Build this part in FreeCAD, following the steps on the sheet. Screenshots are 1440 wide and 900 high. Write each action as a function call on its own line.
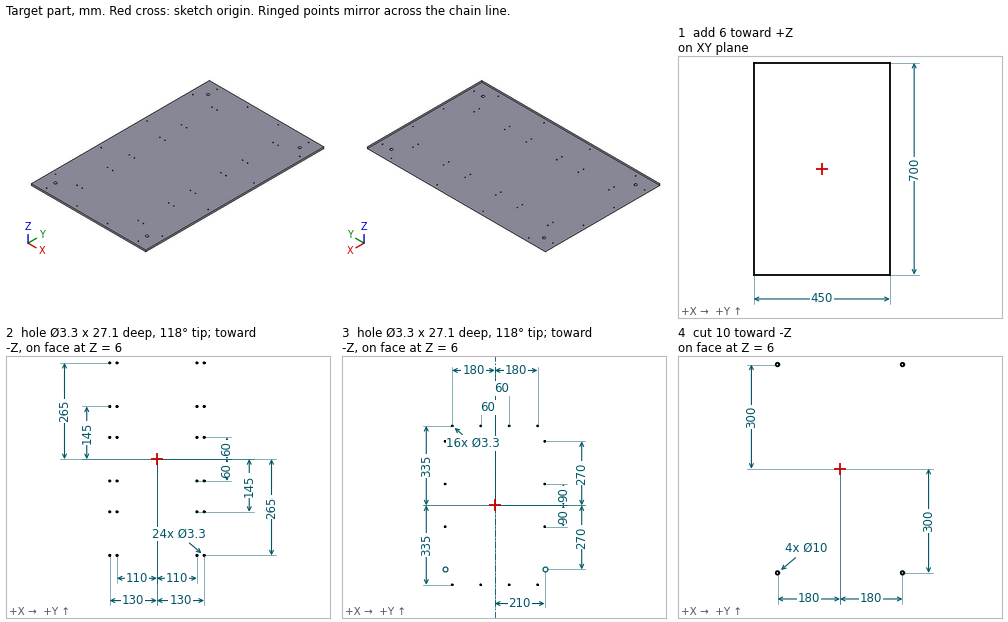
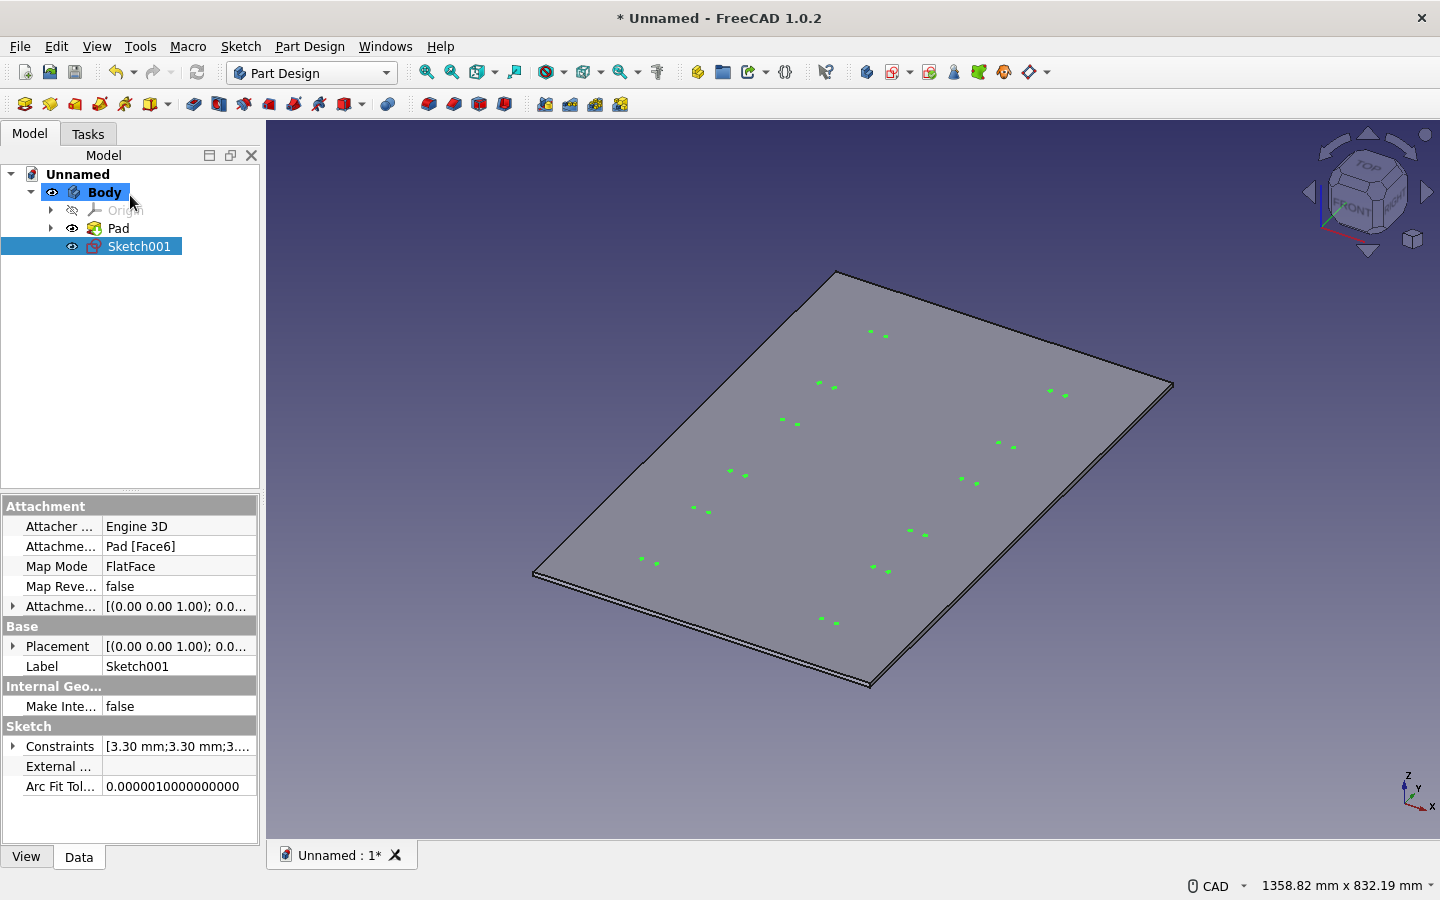
click(219, 104)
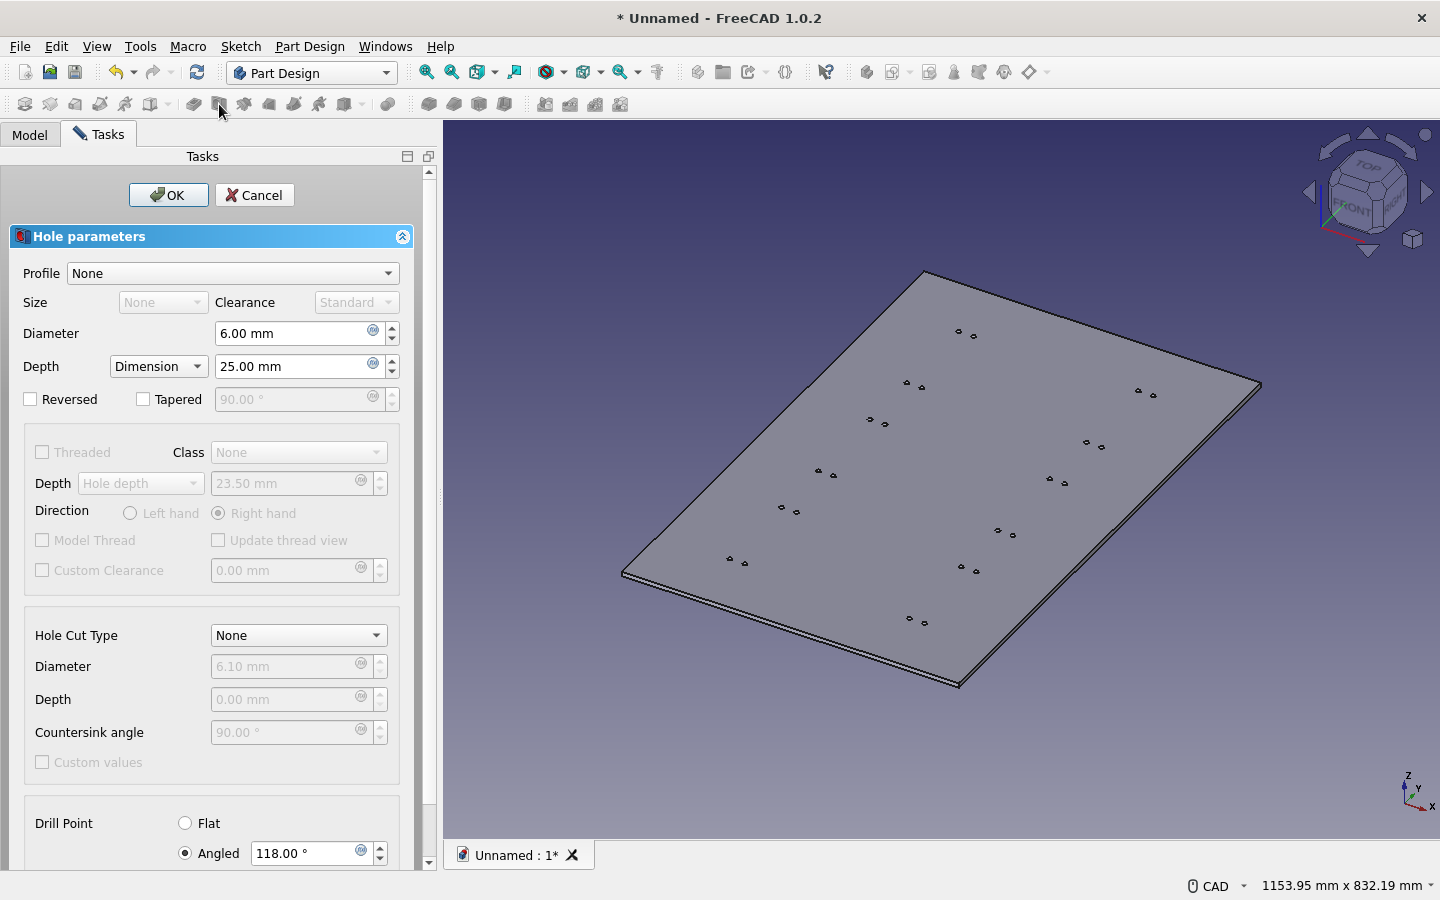
triple_click(300, 334)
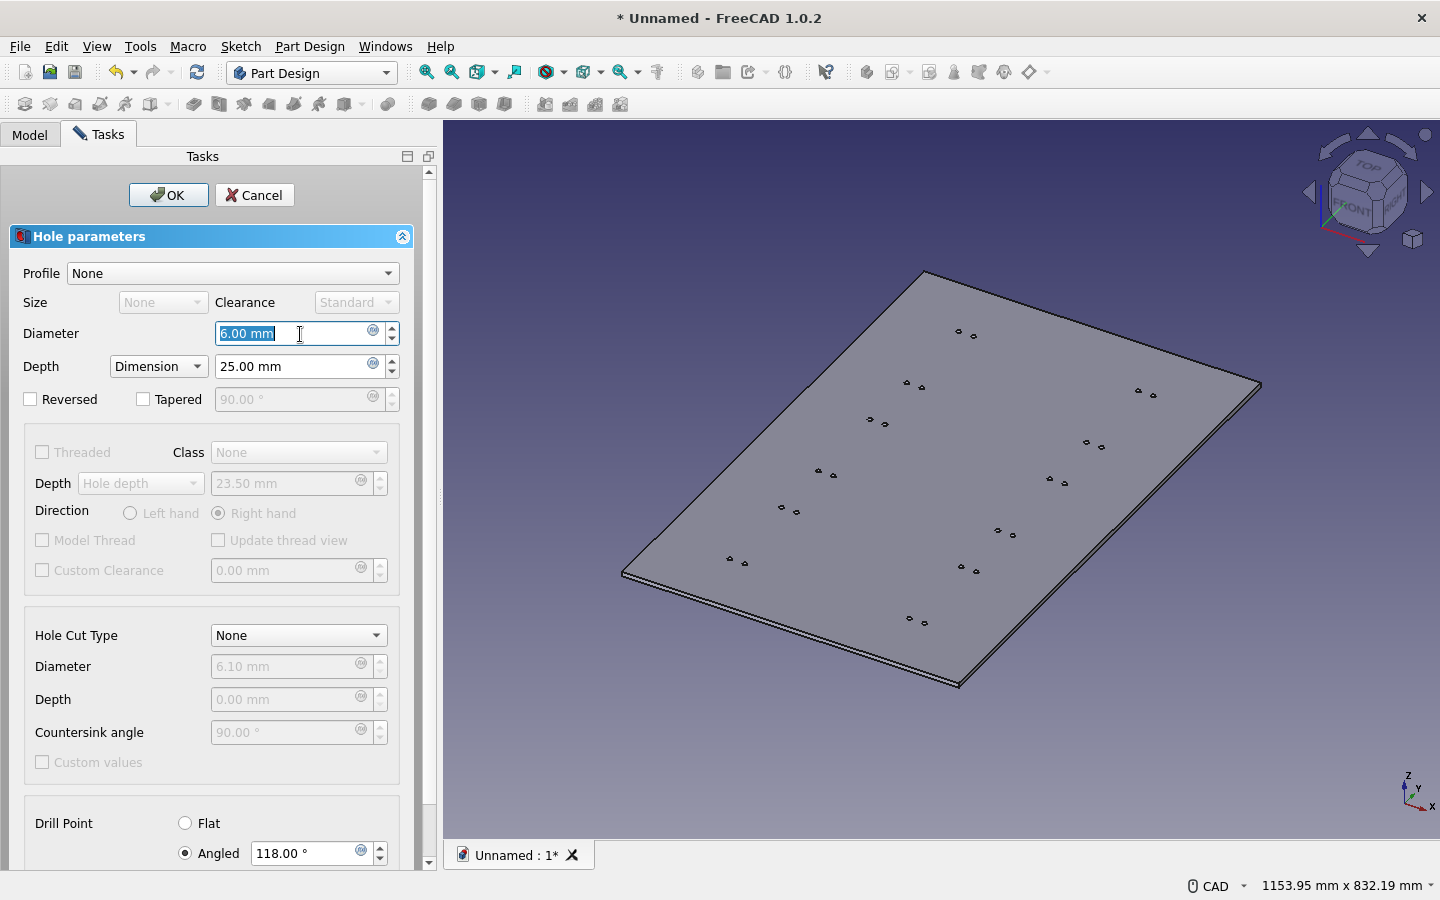
text(3.3)
key(Tab)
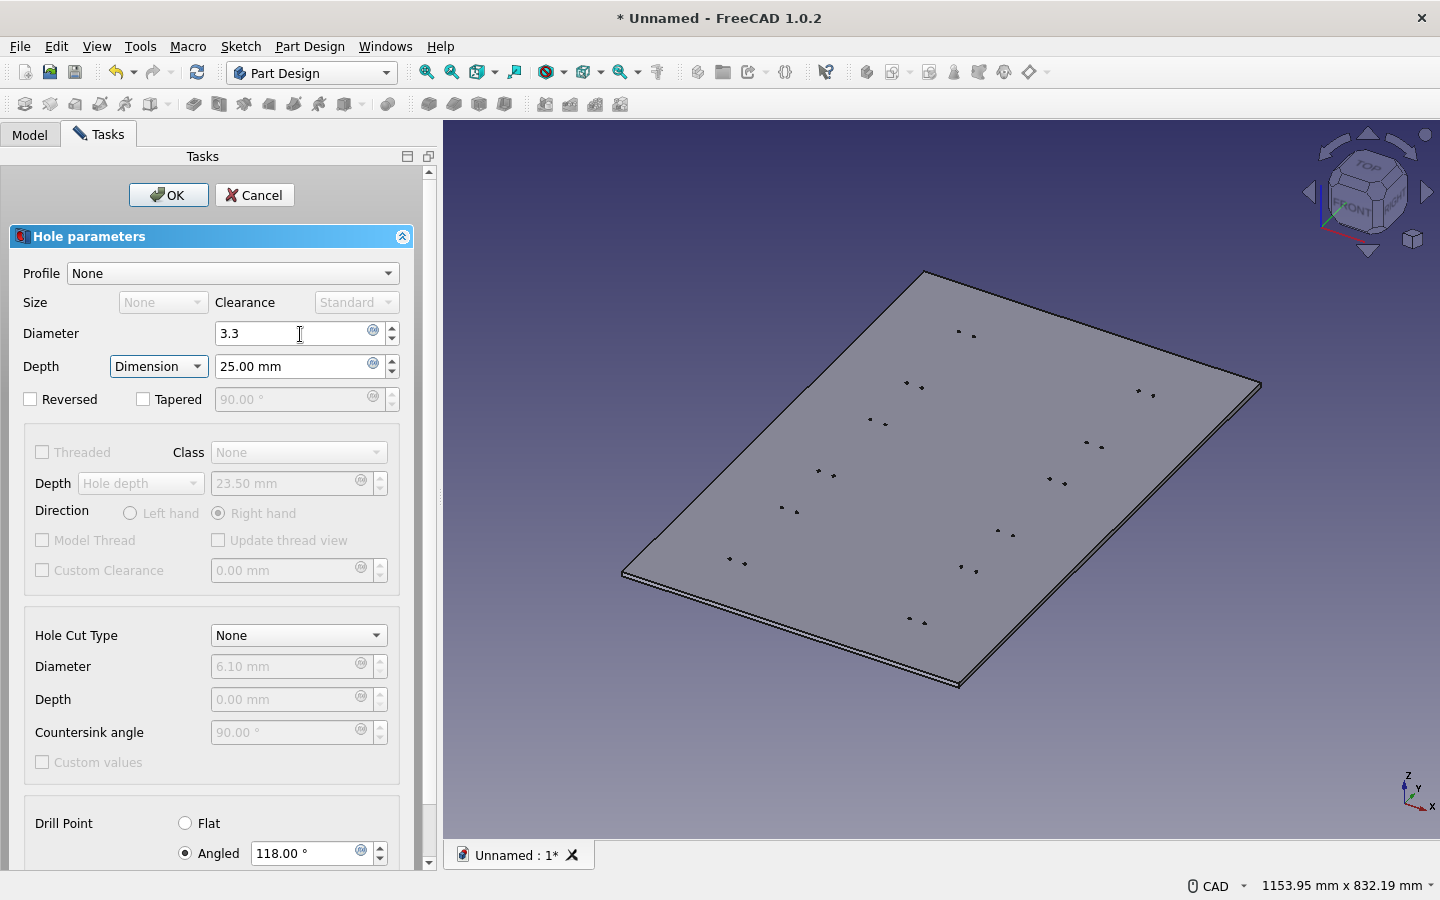
triple_click(300, 366)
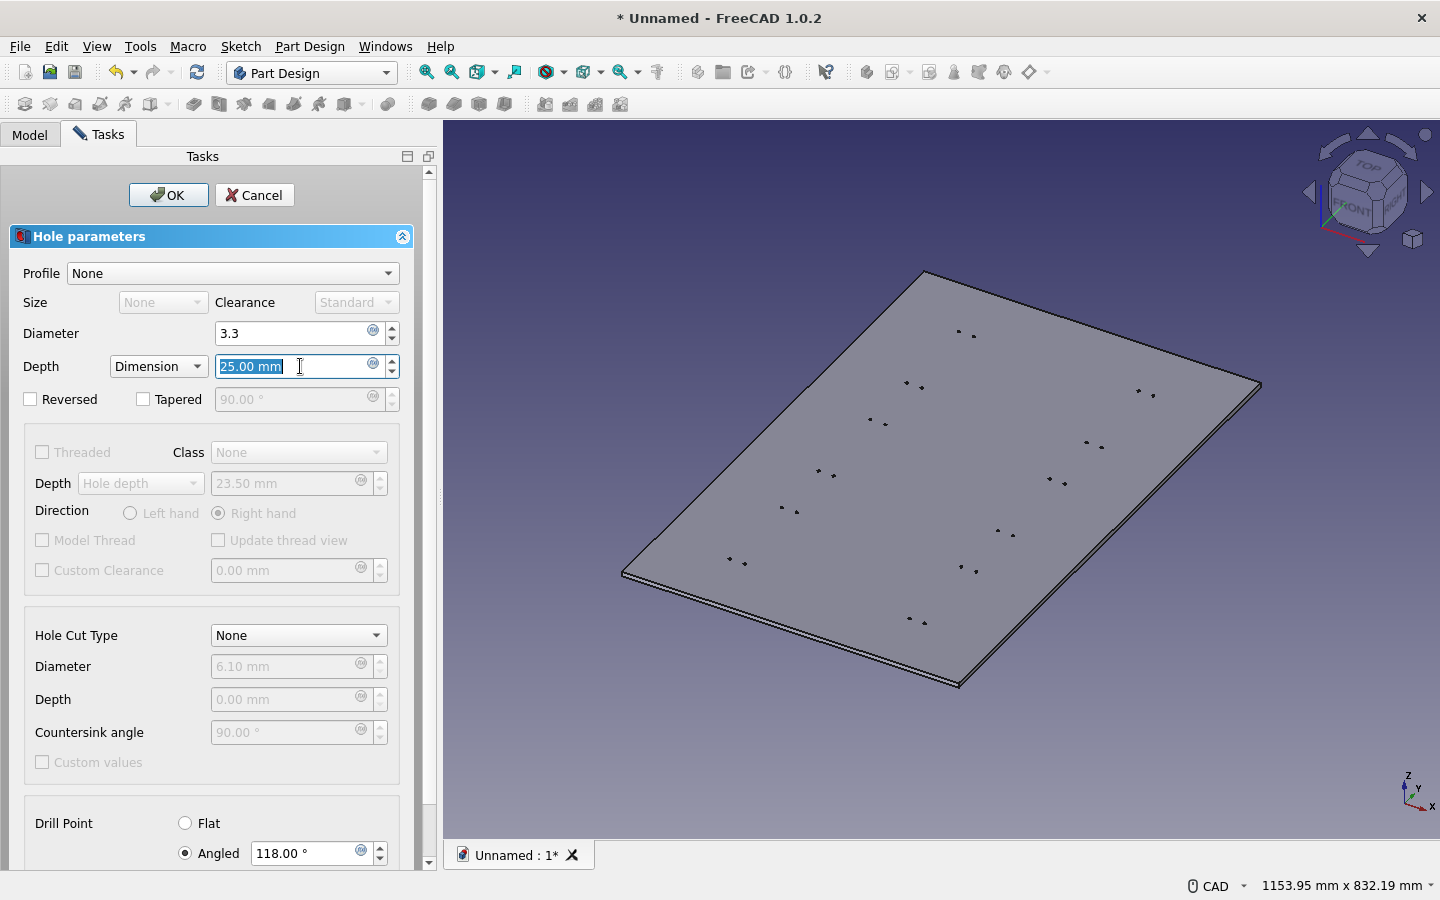
text(27.1)
key(Tab)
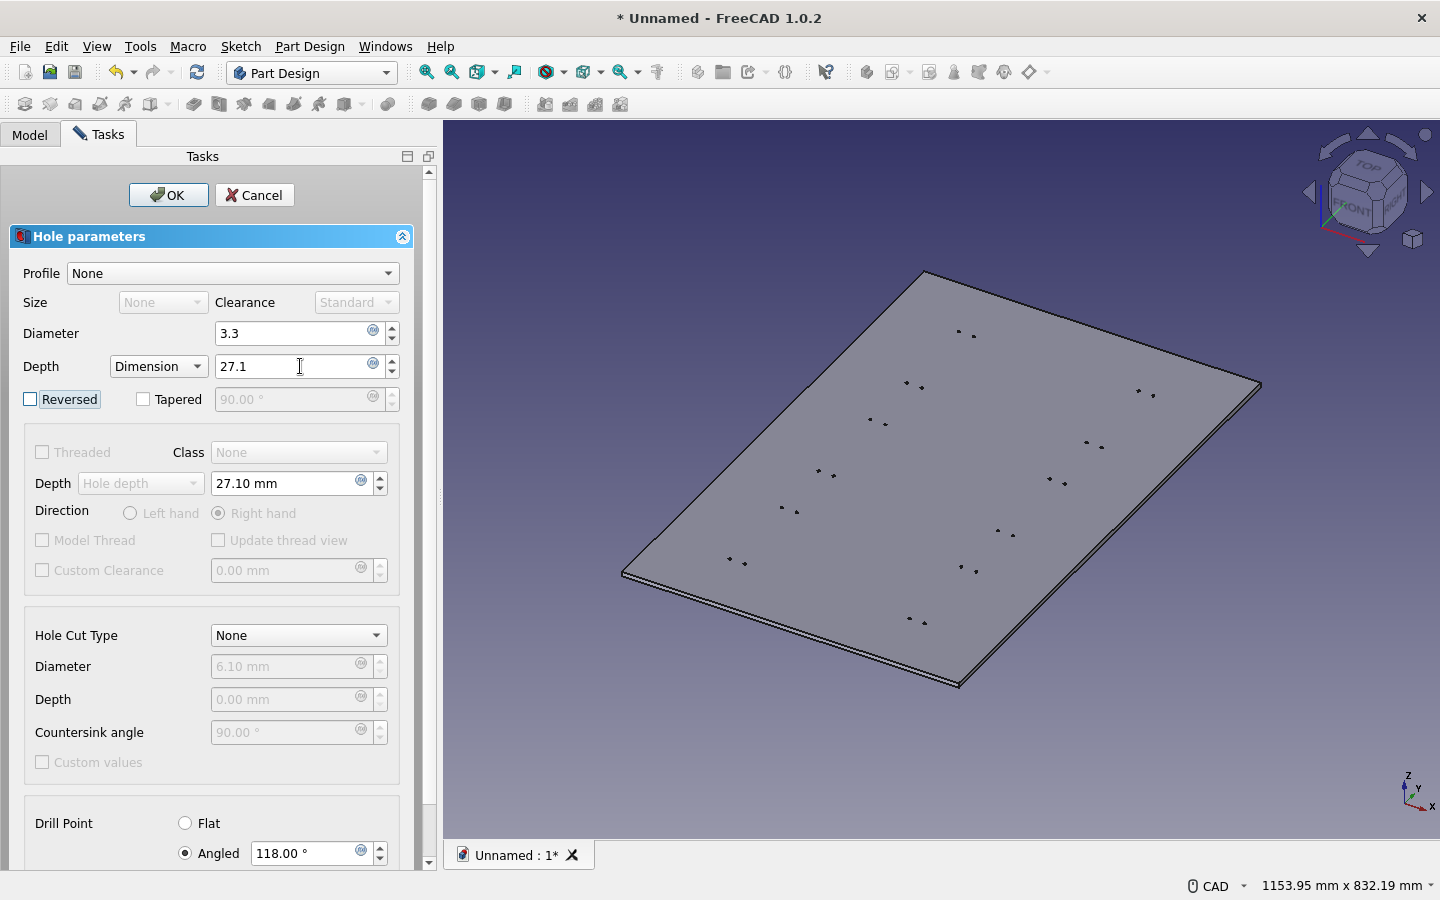
click(169, 195)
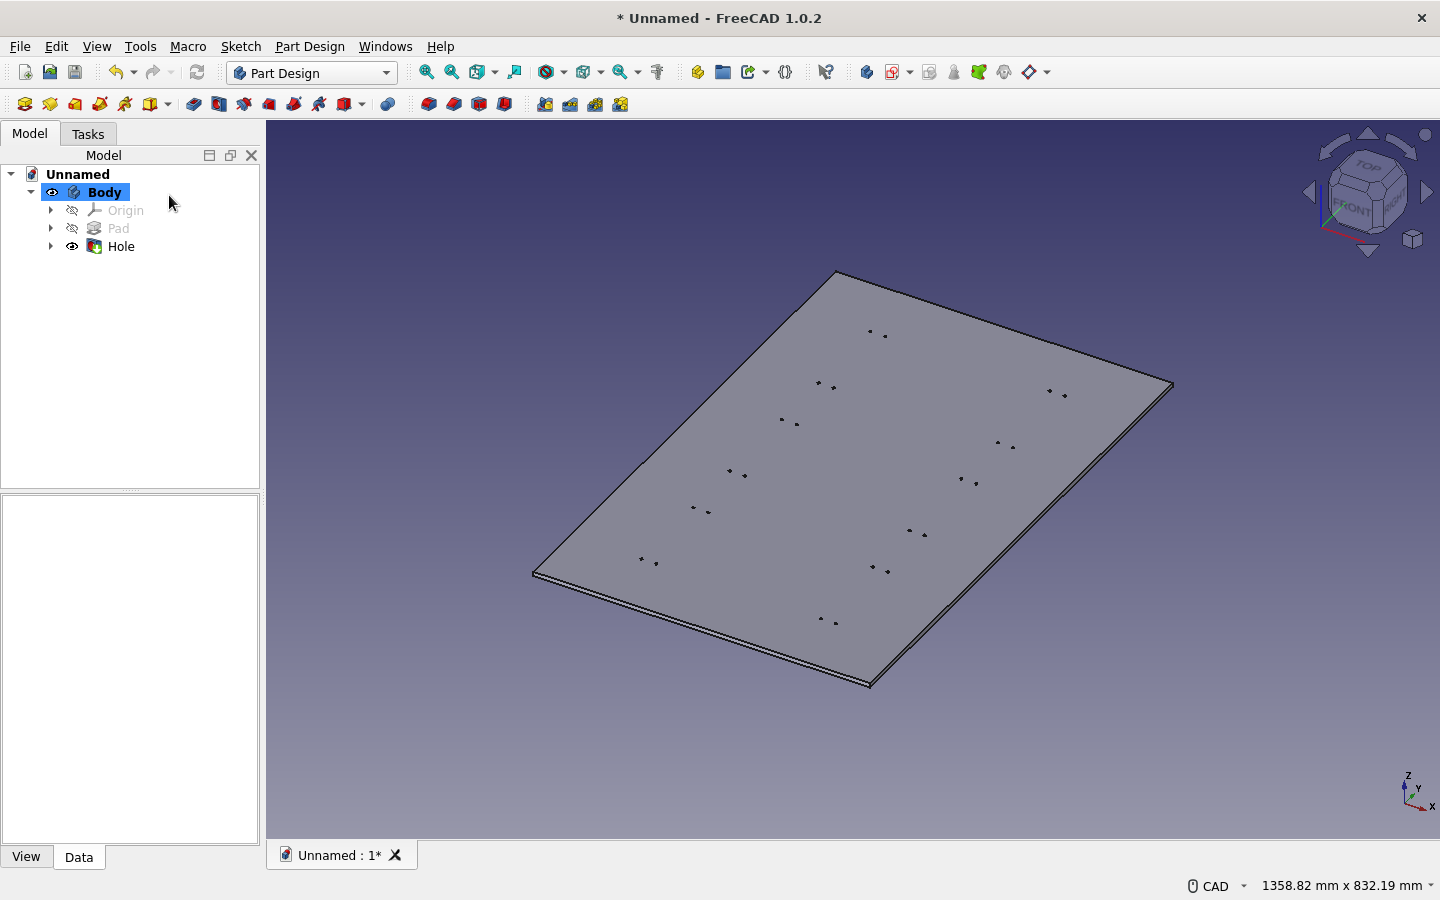
click(853, 476)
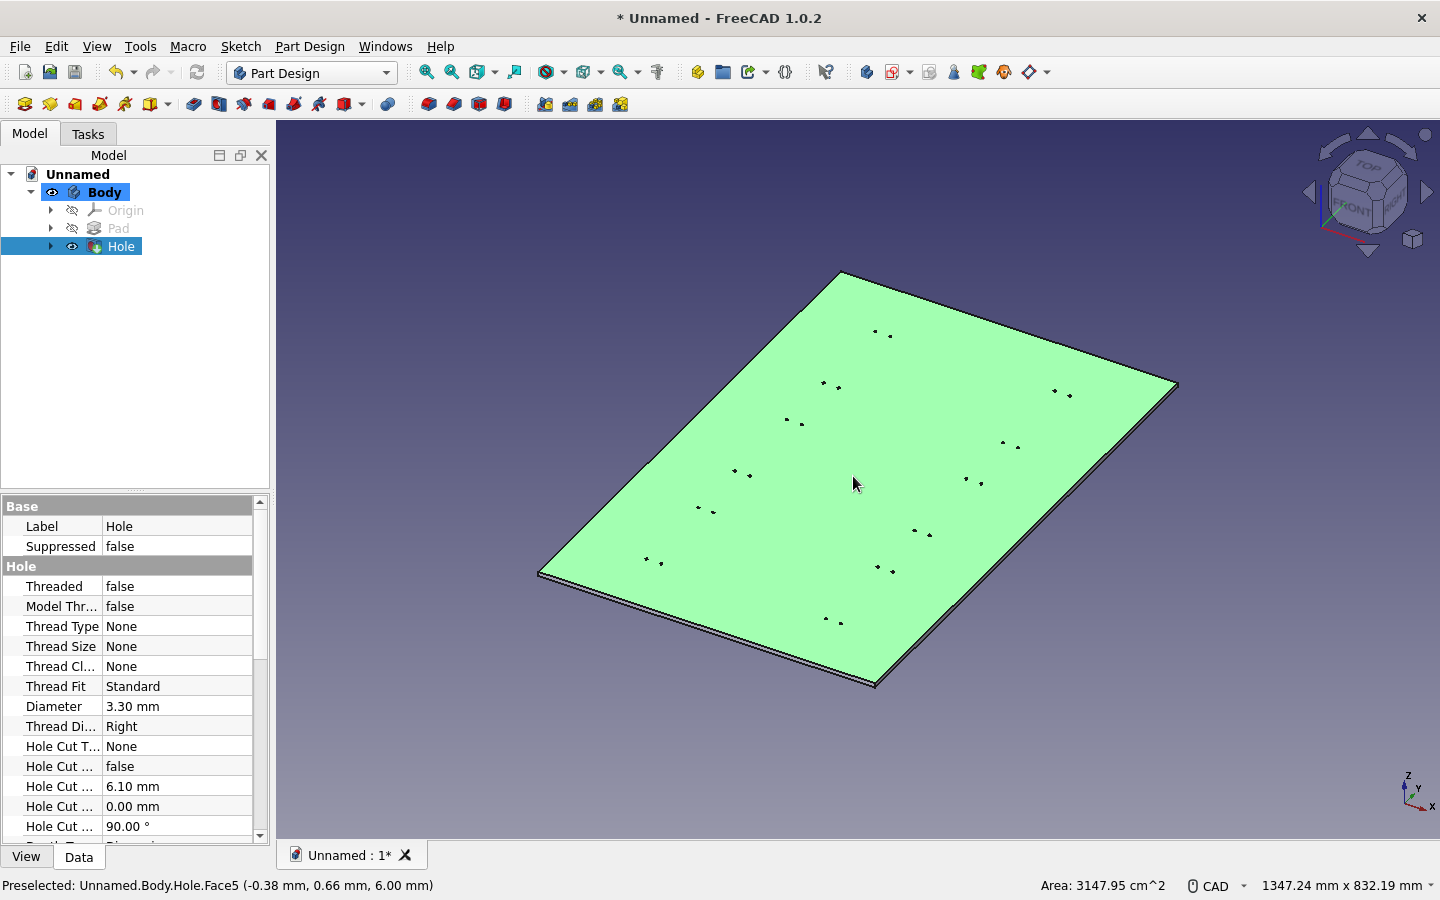
click(892, 72)